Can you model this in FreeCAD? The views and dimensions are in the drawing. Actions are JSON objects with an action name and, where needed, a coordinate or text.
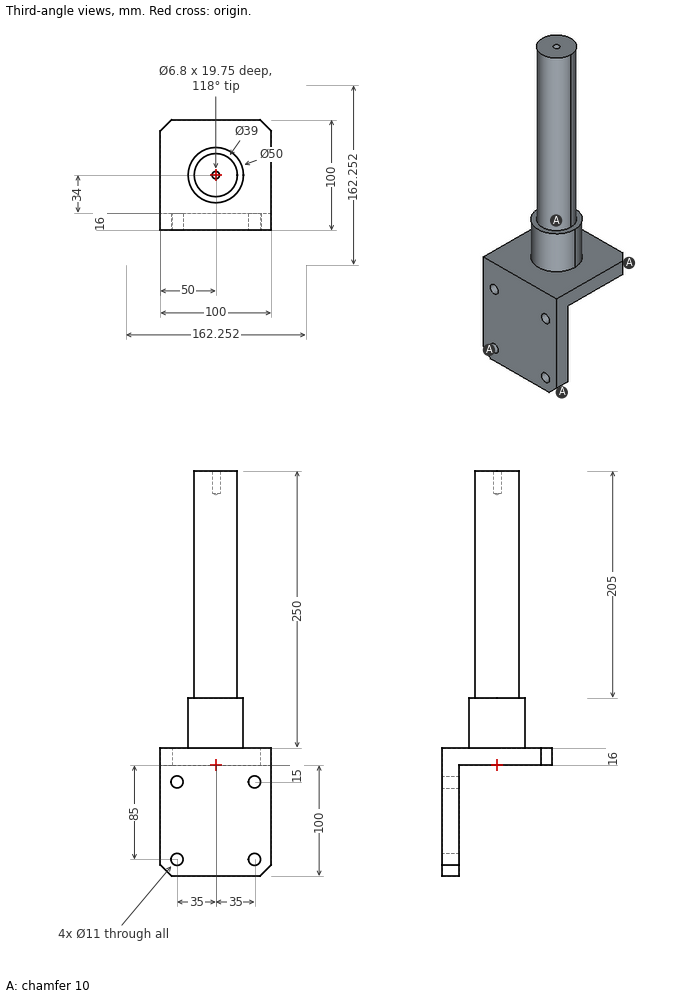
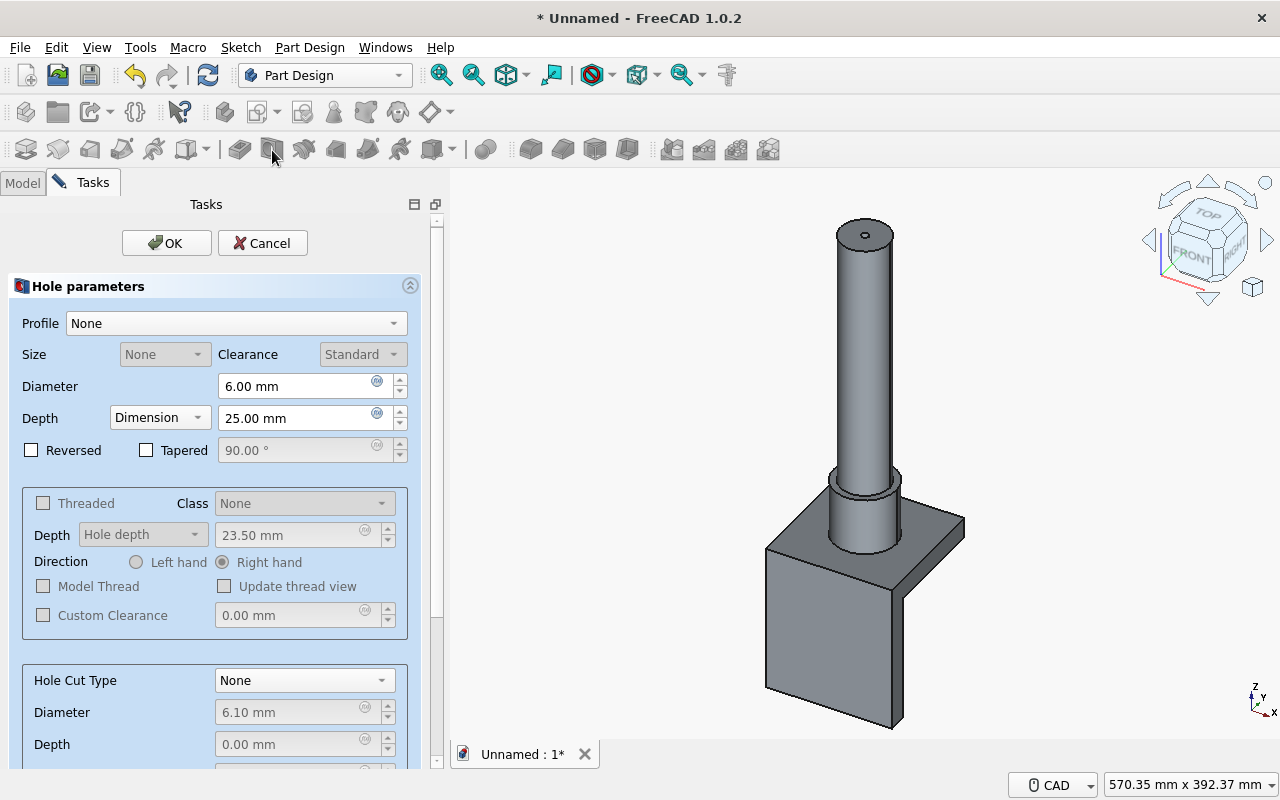
{"action": "triple_click", "coordinate": [305, 386]}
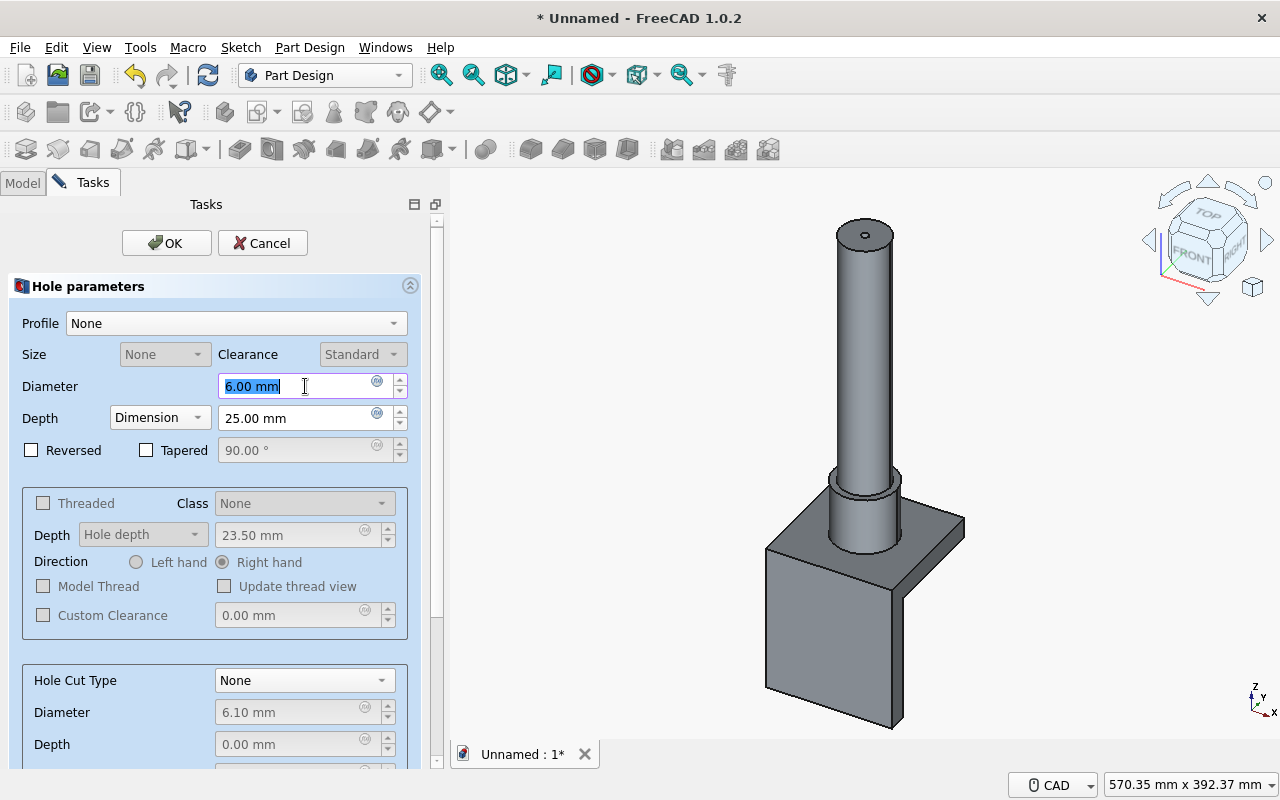
{"action": "type", "text": "6.8"}
{"action": "key", "text": "Tab"}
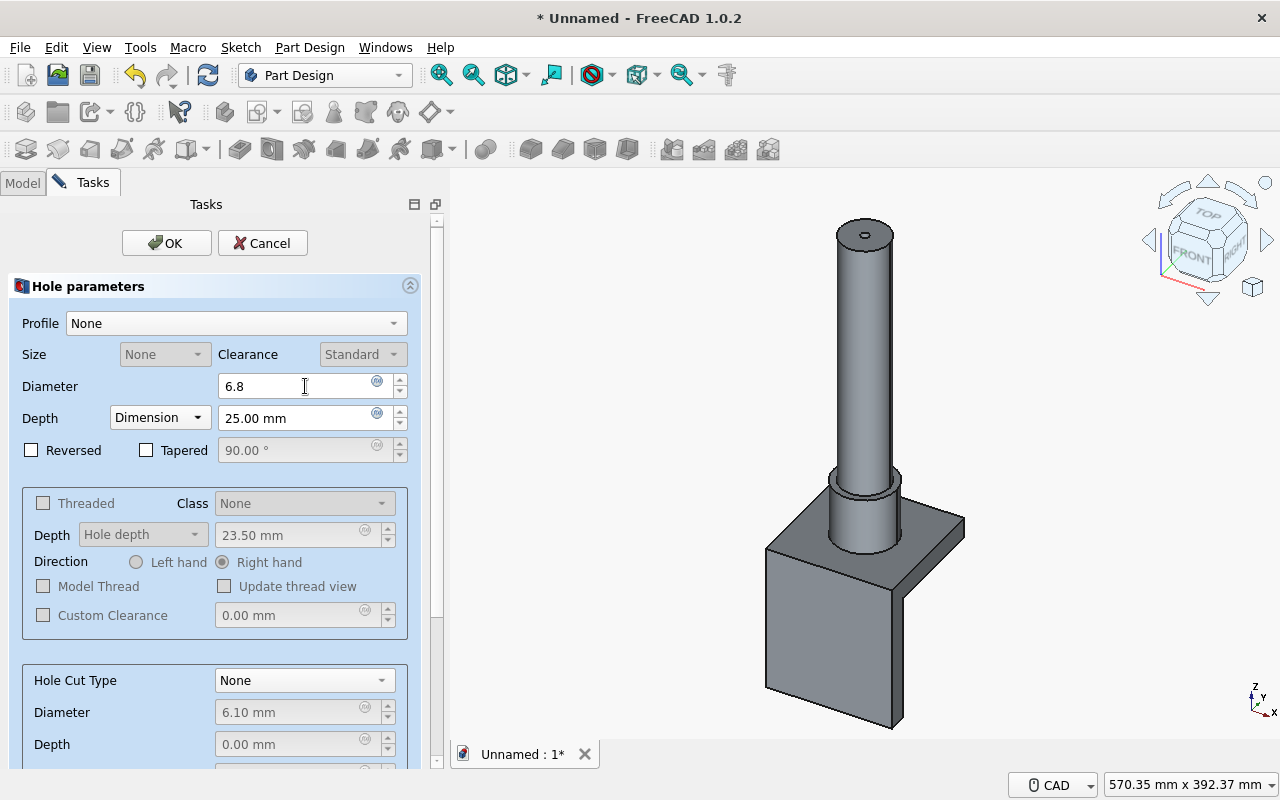
{"action": "triple_click", "coordinate": [305, 418]}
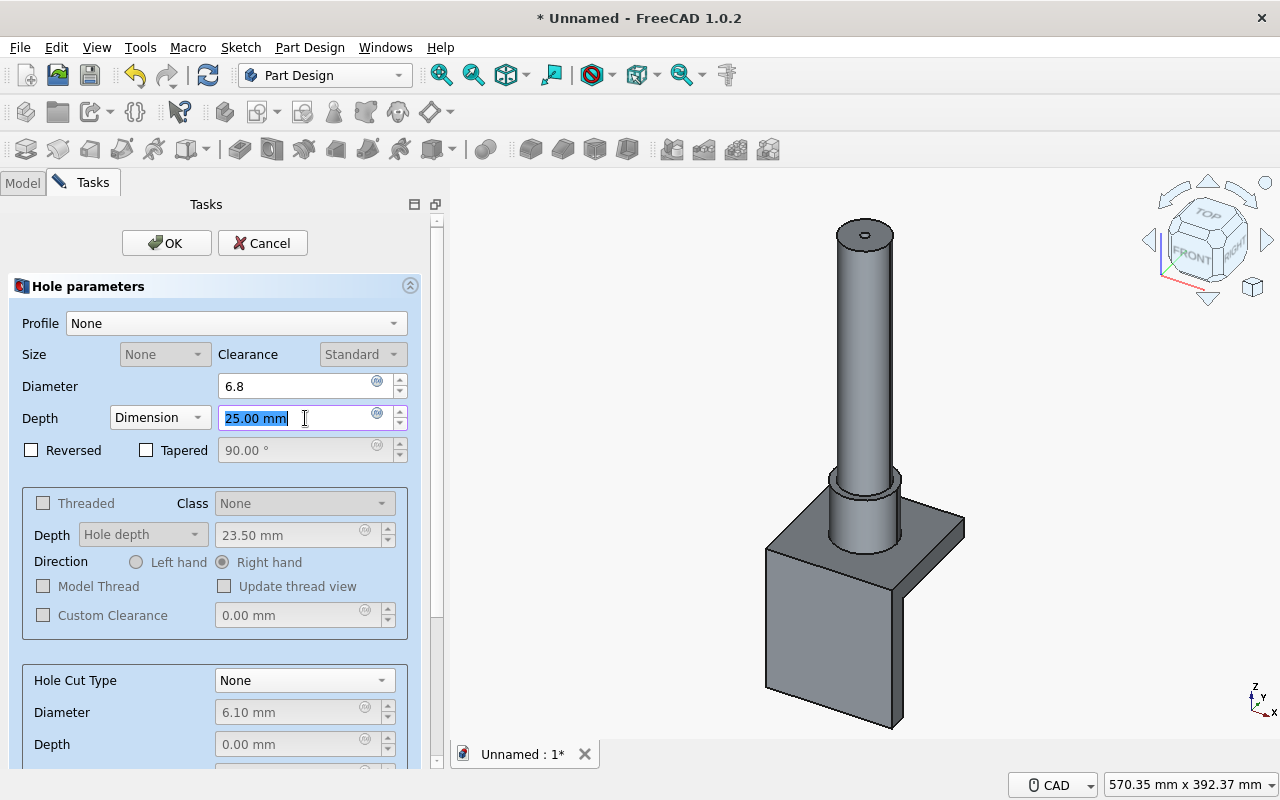
{"action": "type", "text": "19.75"}
{"action": "key", "text": "Tab"}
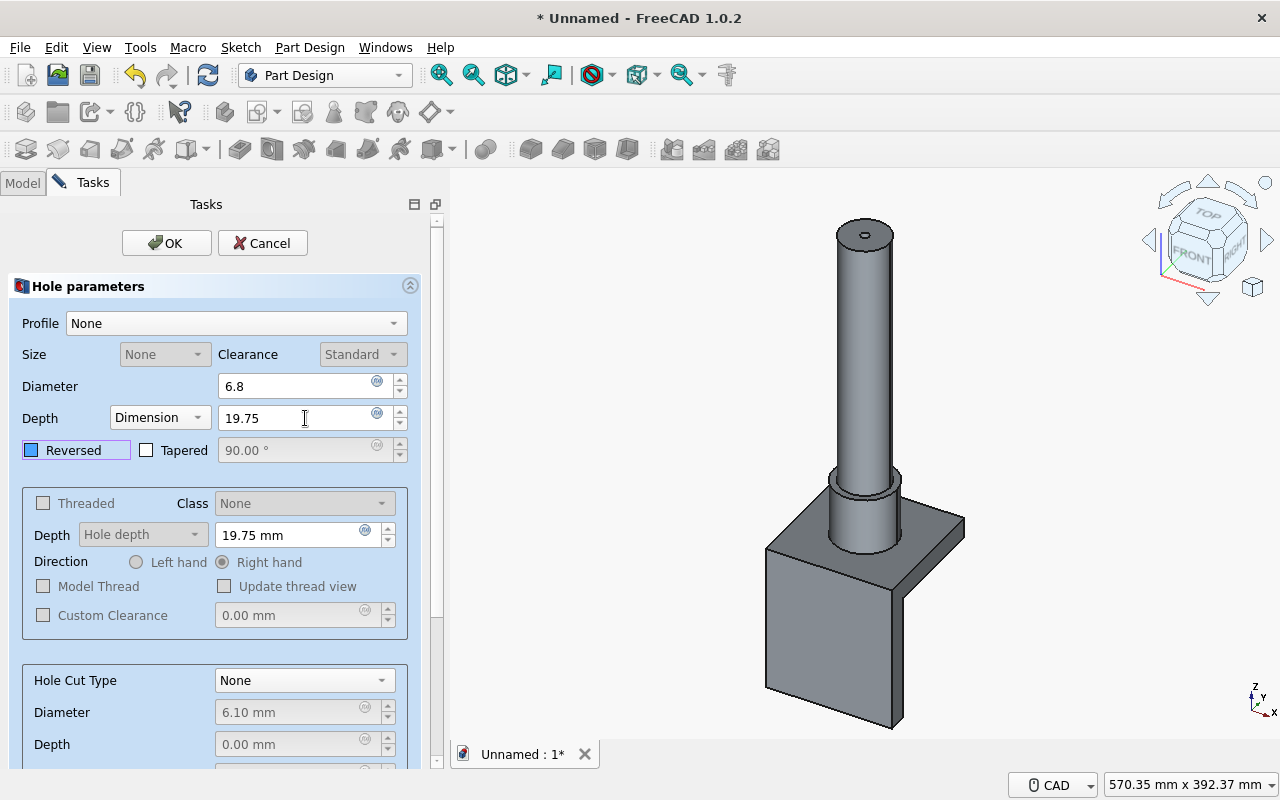
{"action": "left_click", "coordinate": [167, 243]}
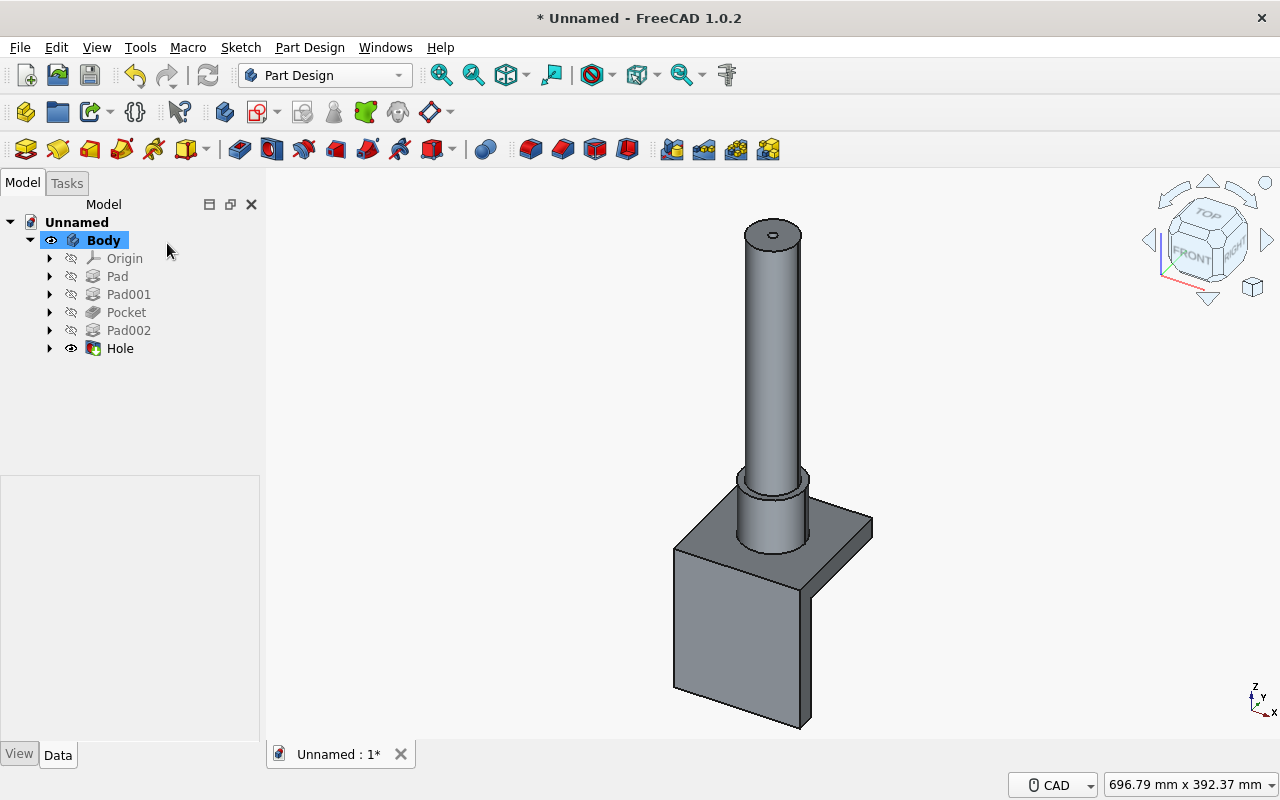
{"action": "key", "text": "4"}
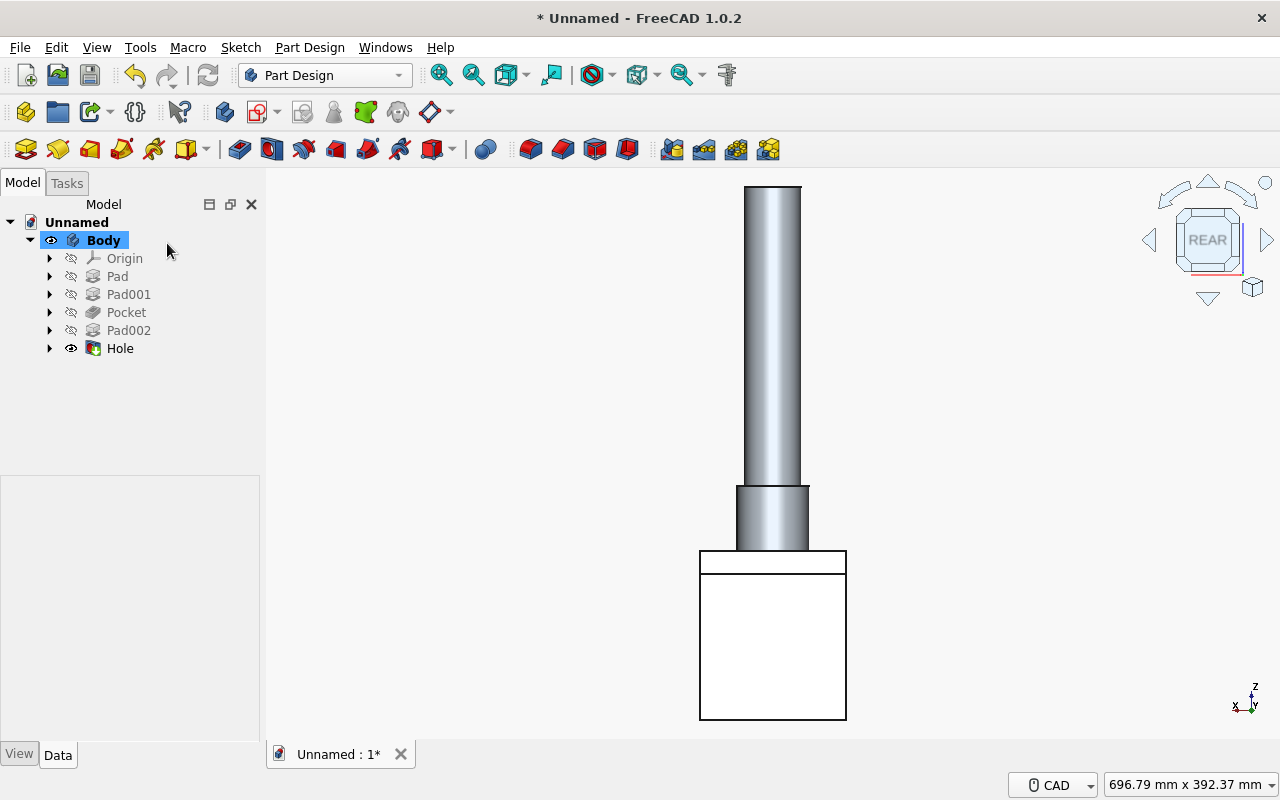
{"action": "left_click", "coordinate": [773, 646]}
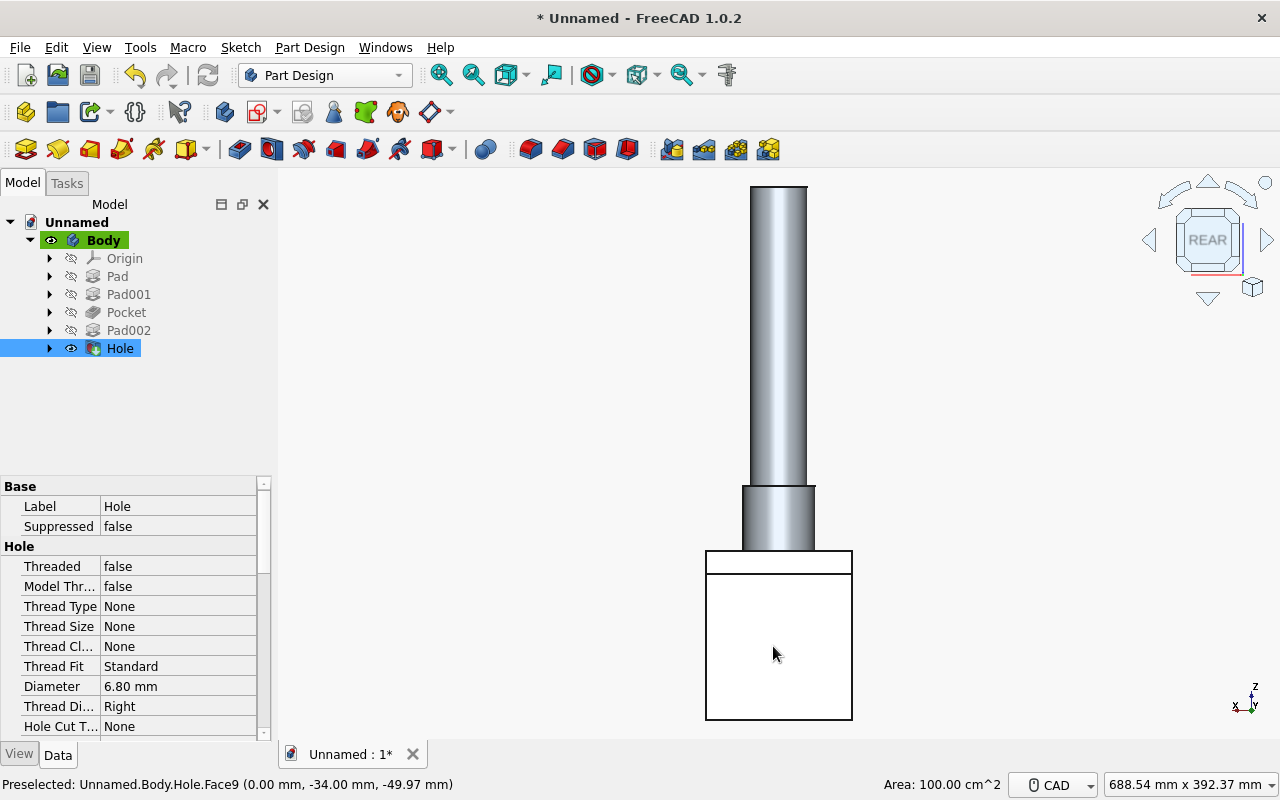
{"action": "left_click", "coordinate": [258, 112]}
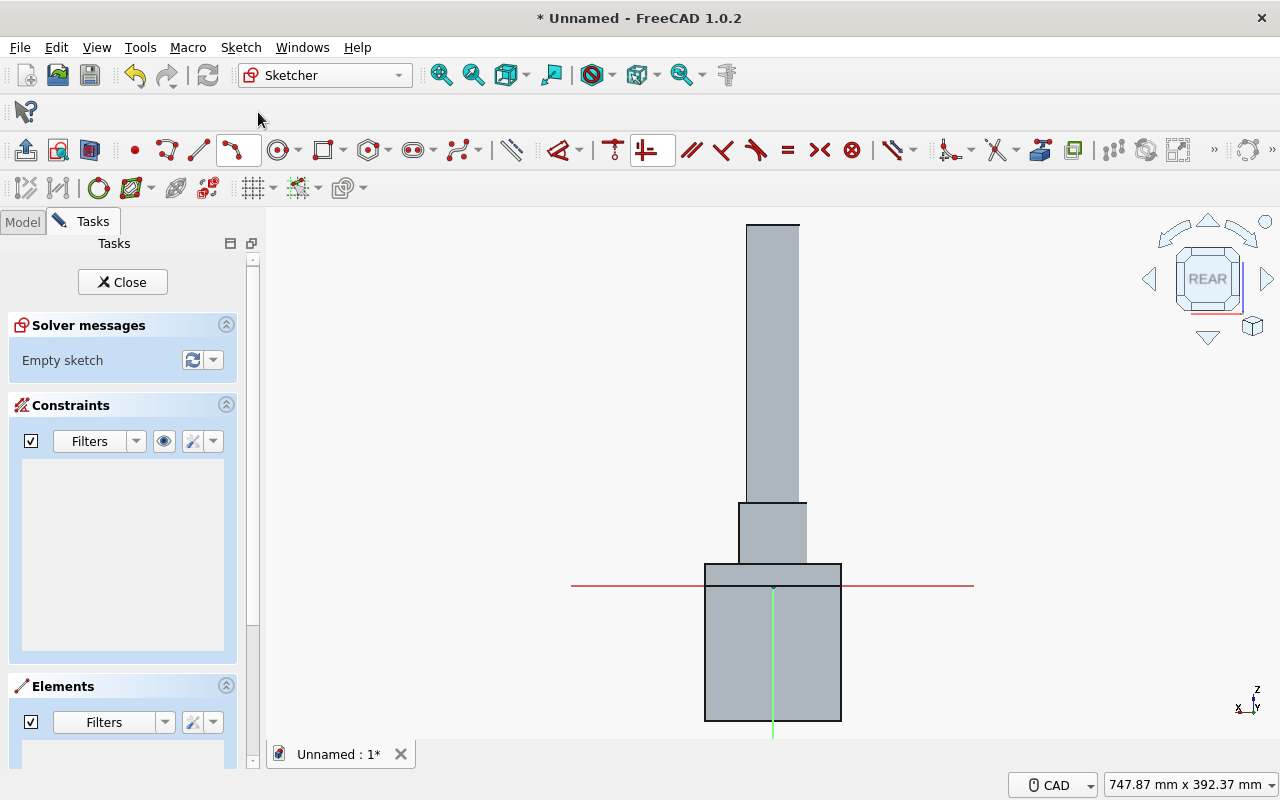
{"action": "left_click", "coordinate": [90, 150]}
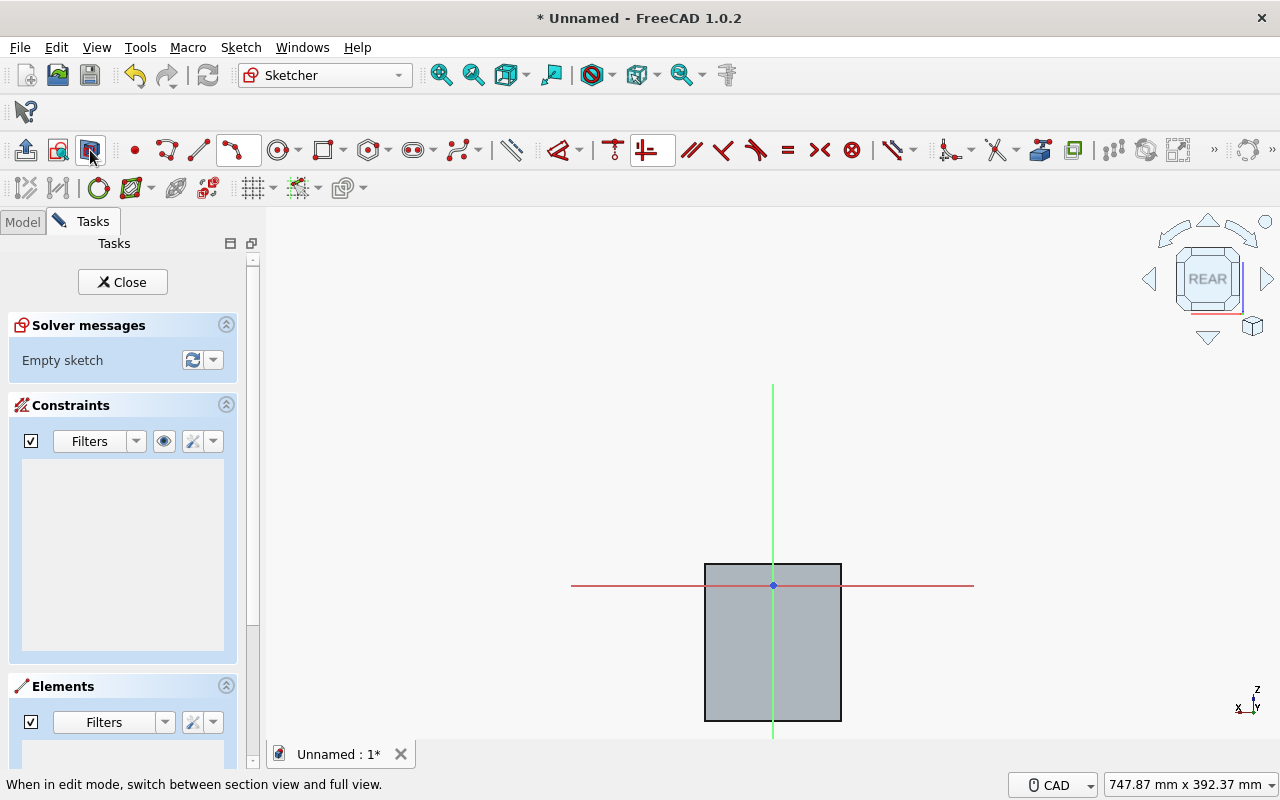
{"action": "scroll", "coordinate": [704, 473], "scroll_direction": "down", "scroll_amount": 5}